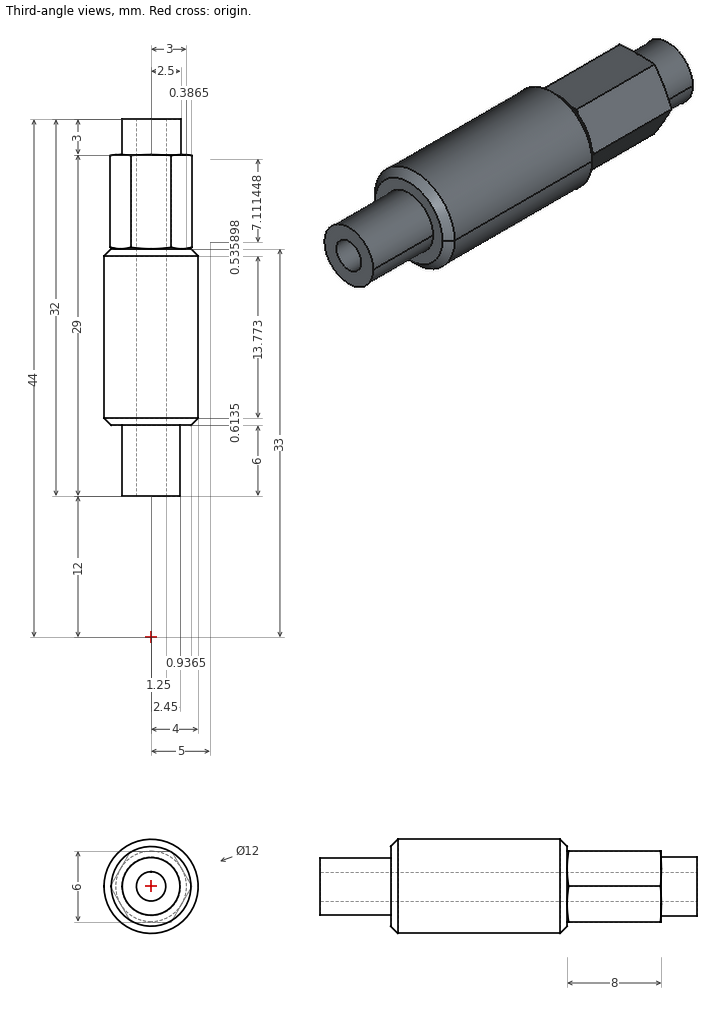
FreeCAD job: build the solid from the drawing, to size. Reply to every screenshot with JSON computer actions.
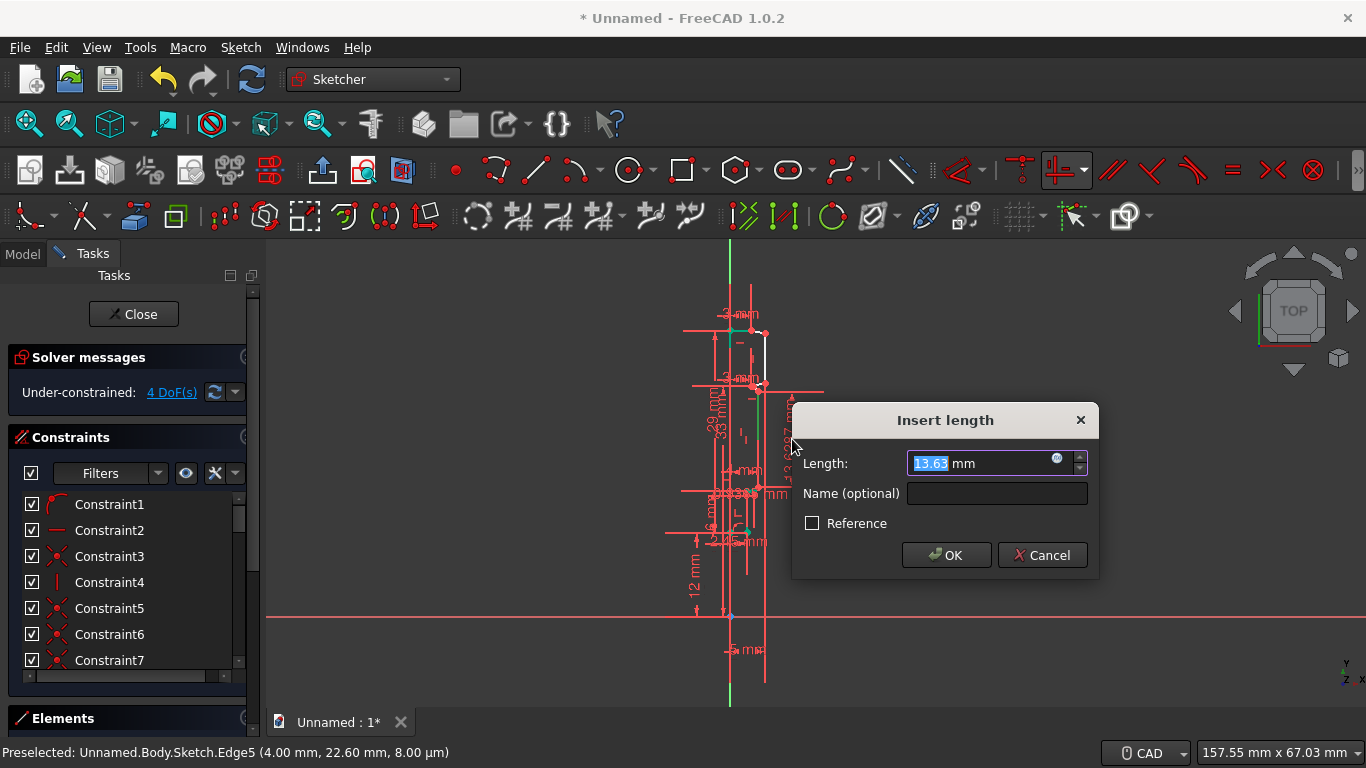
{"action": "type", "text": "13.773"}
{"action": "key", "text": "Return"}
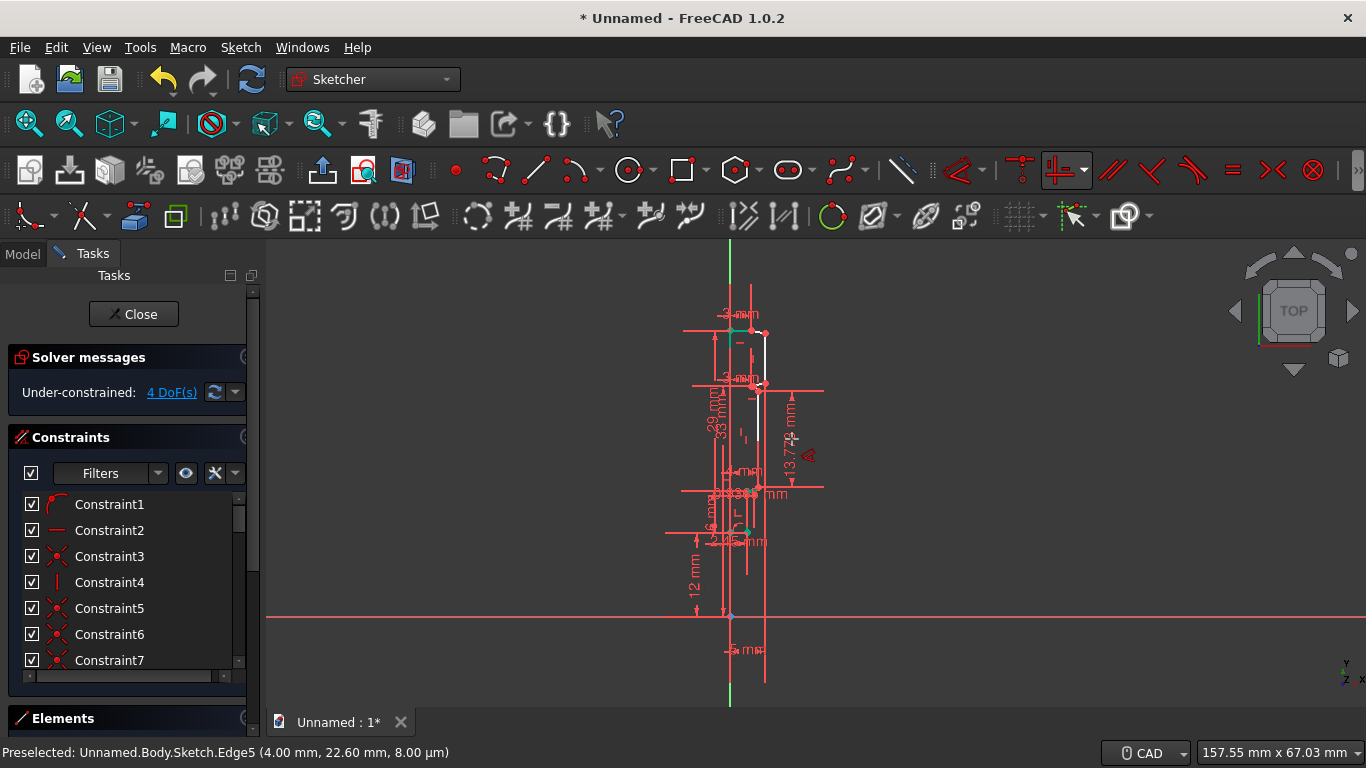
{"action": "scroll", "coordinate": [753, 386], "scroll_direction": "up", "scroll_amount": 14}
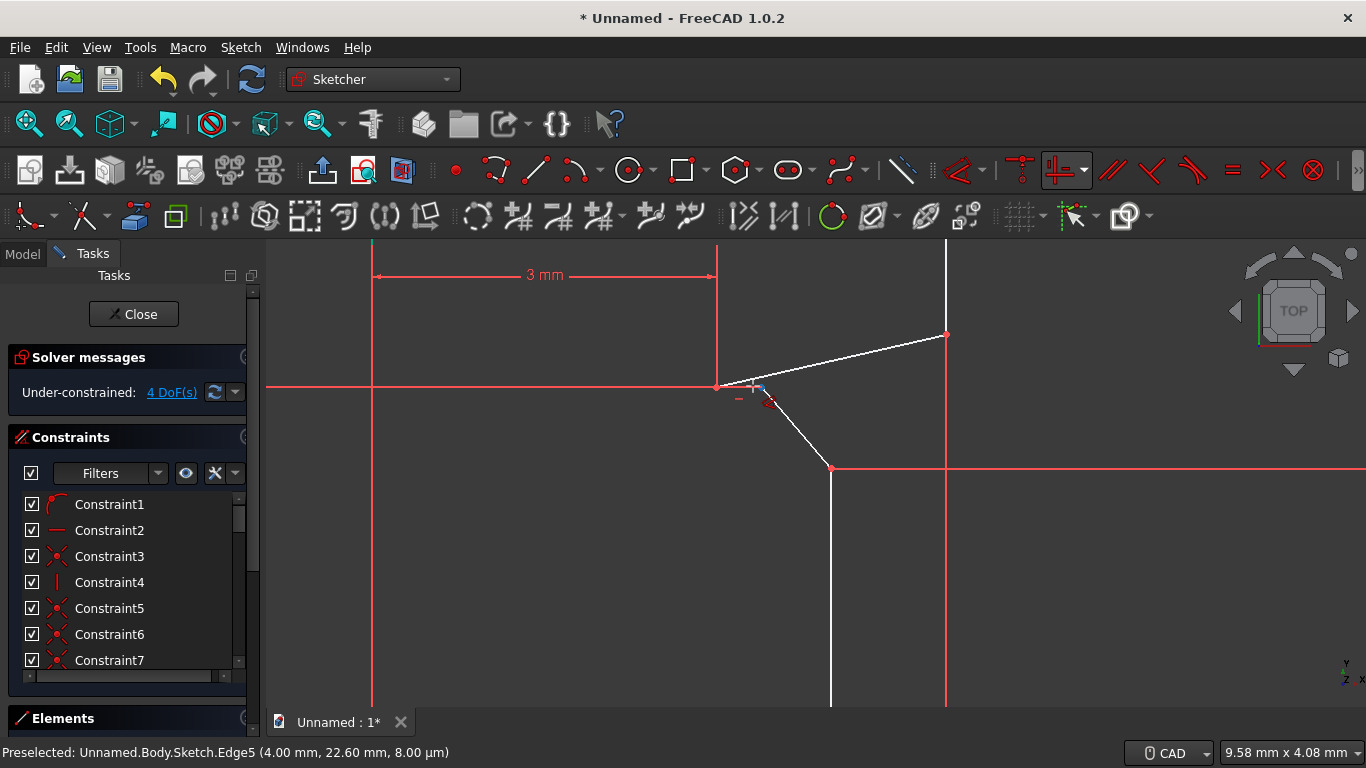
{"action": "left_click", "coordinate": [753, 387]}
{"action": "left_click", "coordinate": [739, 353]}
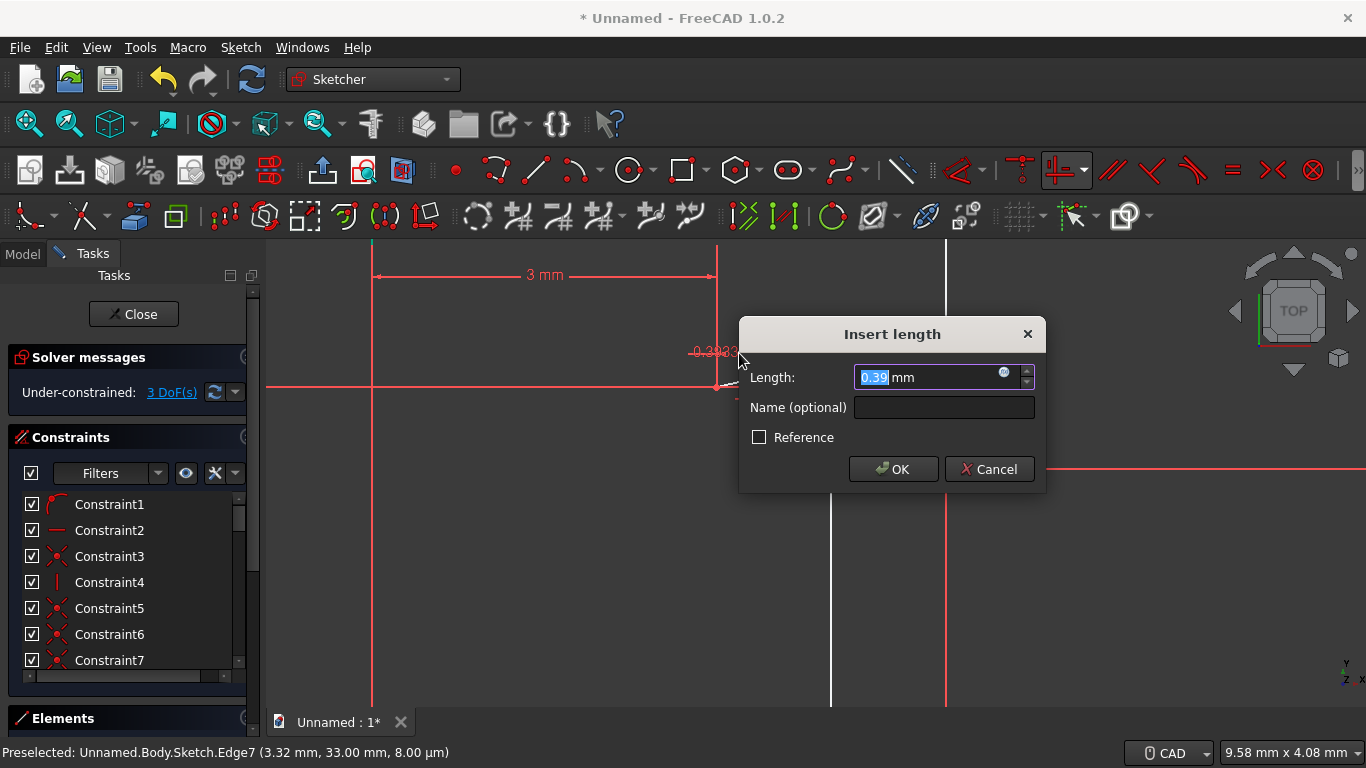
{"action": "type", "text": "0.3865"}
{"action": "key", "text": "Return"}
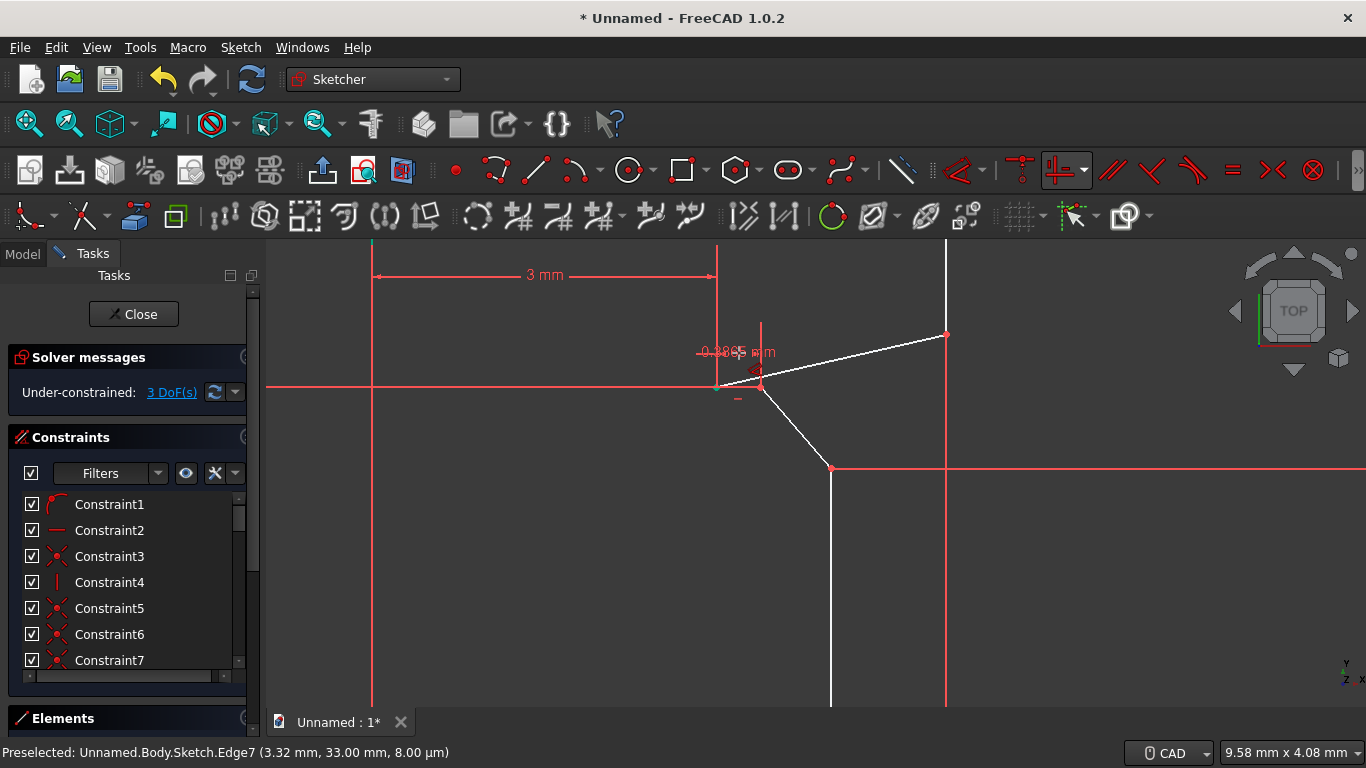
{"action": "scroll", "coordinate": [753, 386], "scroll_direction": "down", "scroll_amount": 14}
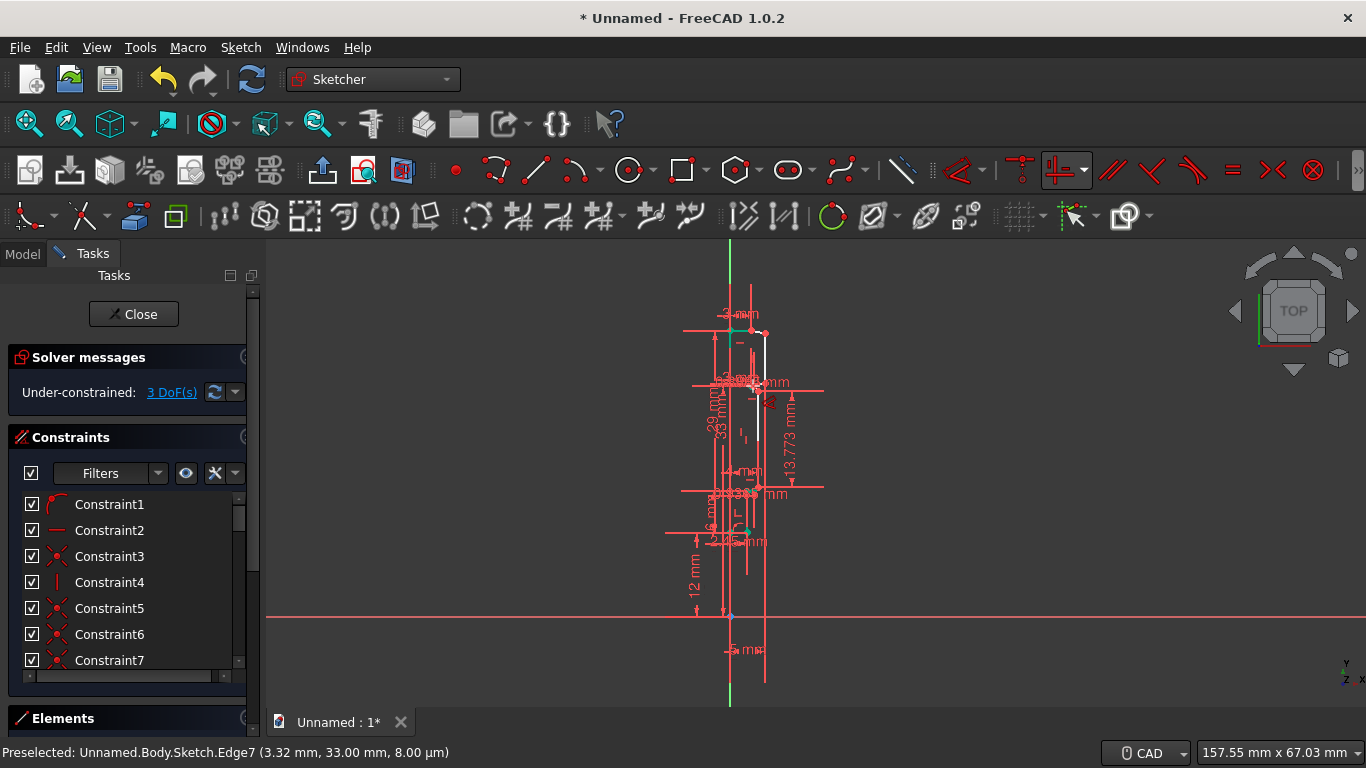
{"action": "scroll", "coordinate": [755, 490], "scroll_direction": "up", "scroll_amount": 12}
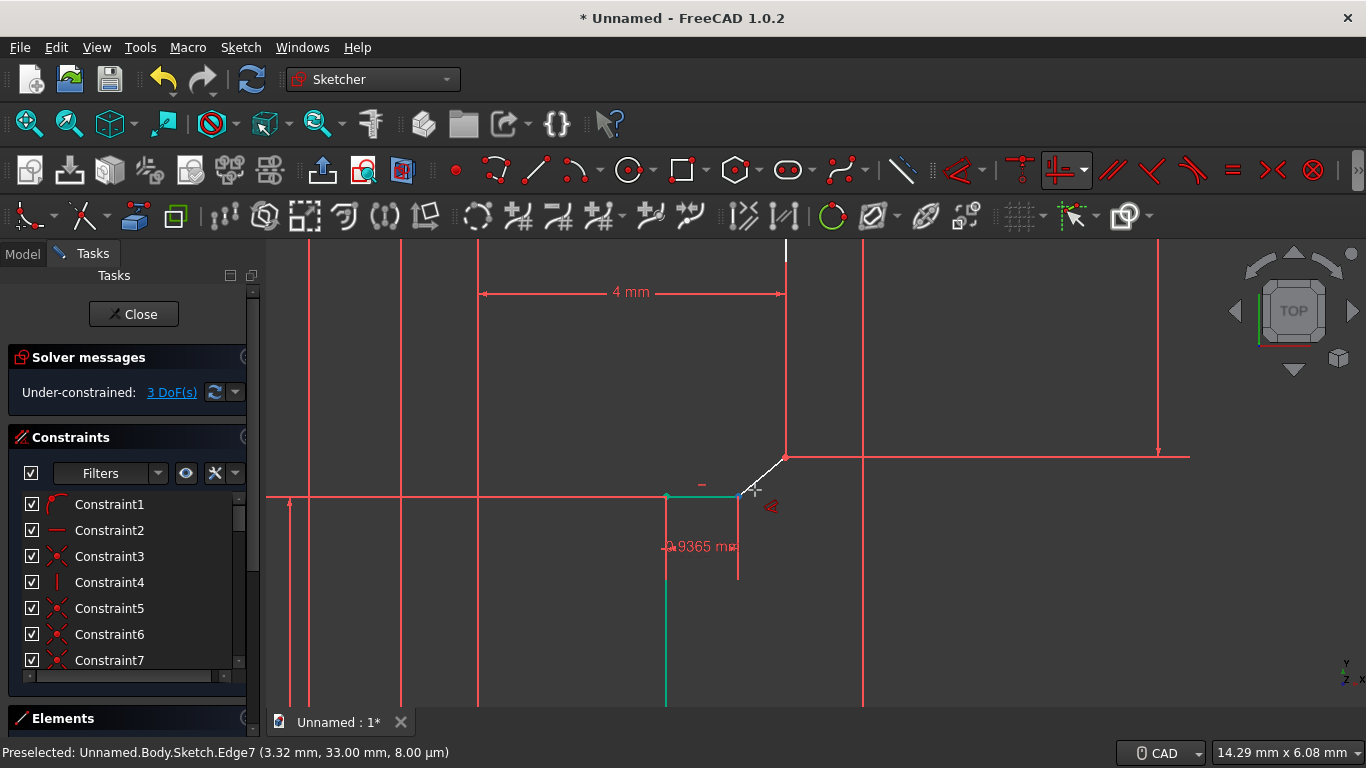
{"action": "left_click", "coordinate": [753, 485]}
{"action": "left_click", "coordinate": [820, 477]}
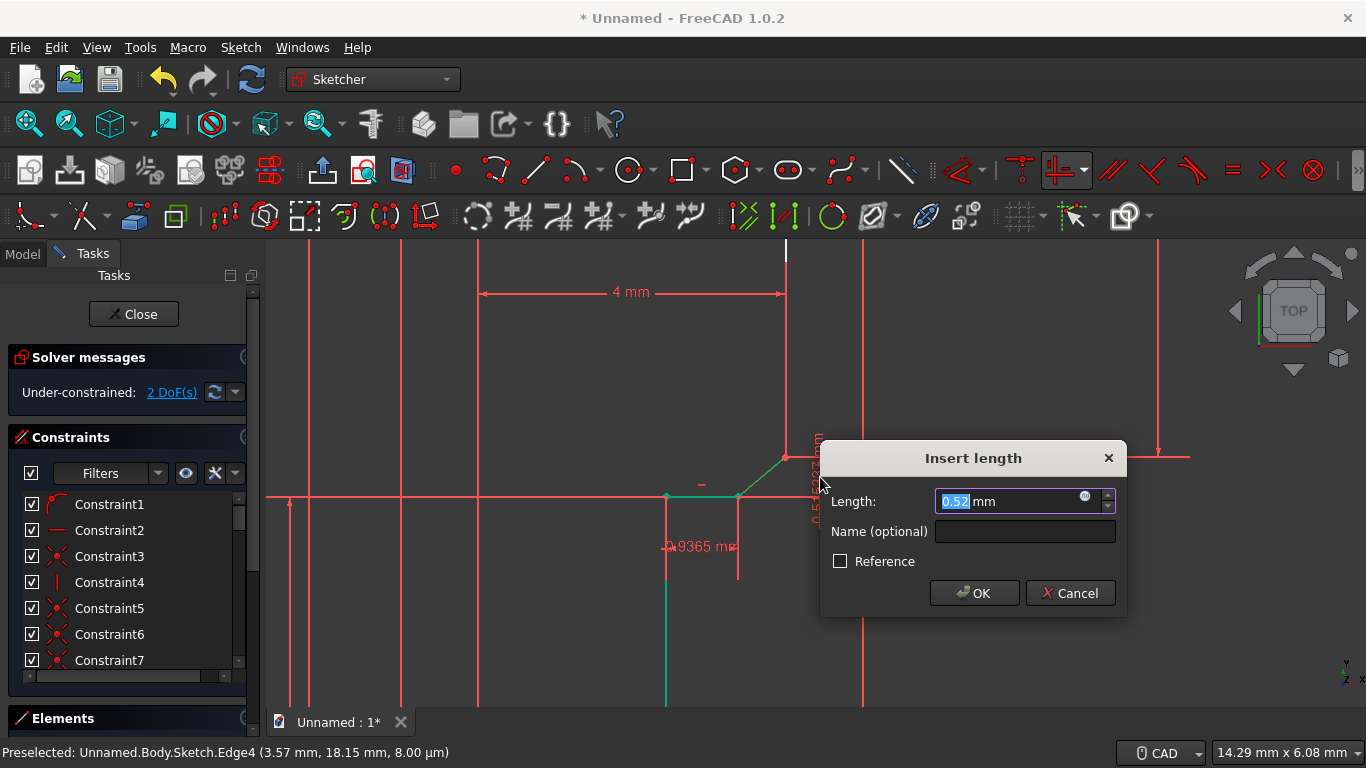
{"action": "type", "text": "0.6135"}
{"action": "key", "text": "Return"}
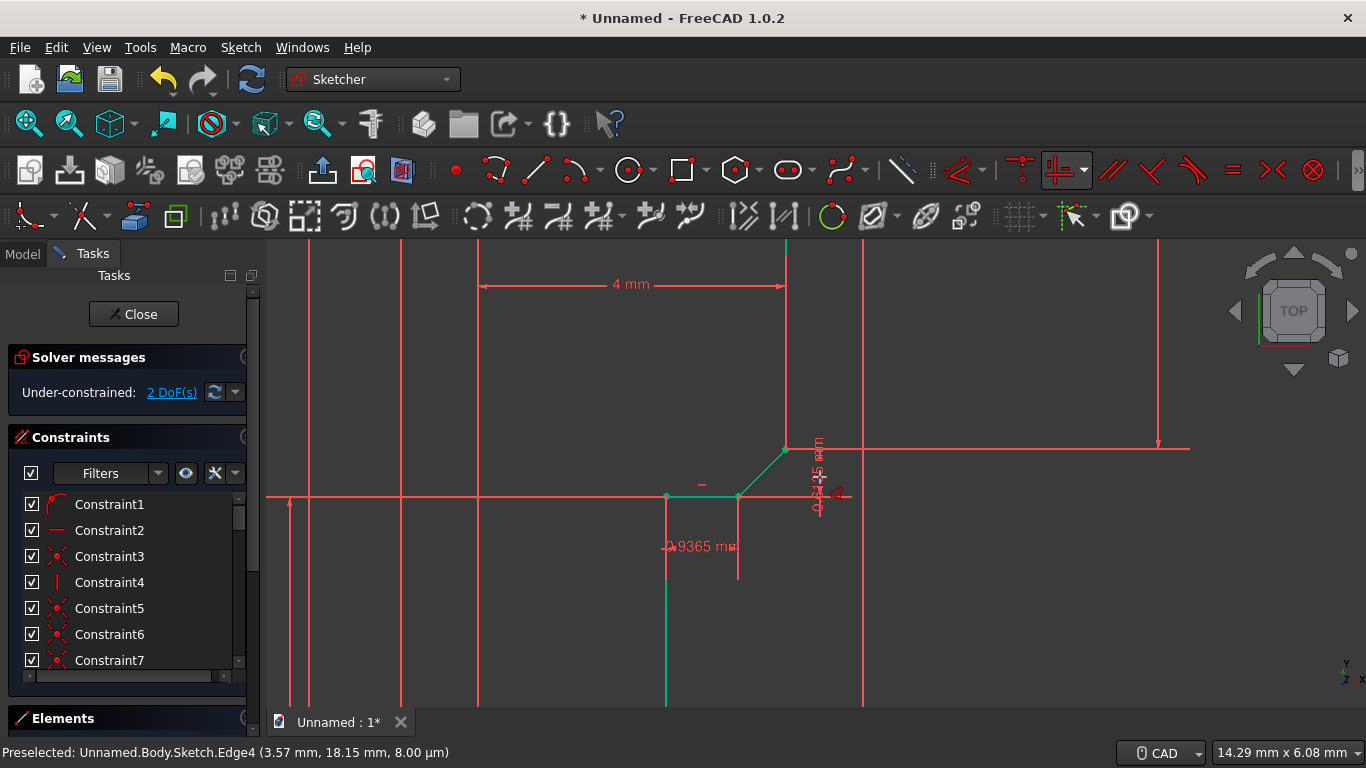
{"action": "scroll", "coordinate": [755, 490], "scroll_direction": "down", "scroll_amount": 12}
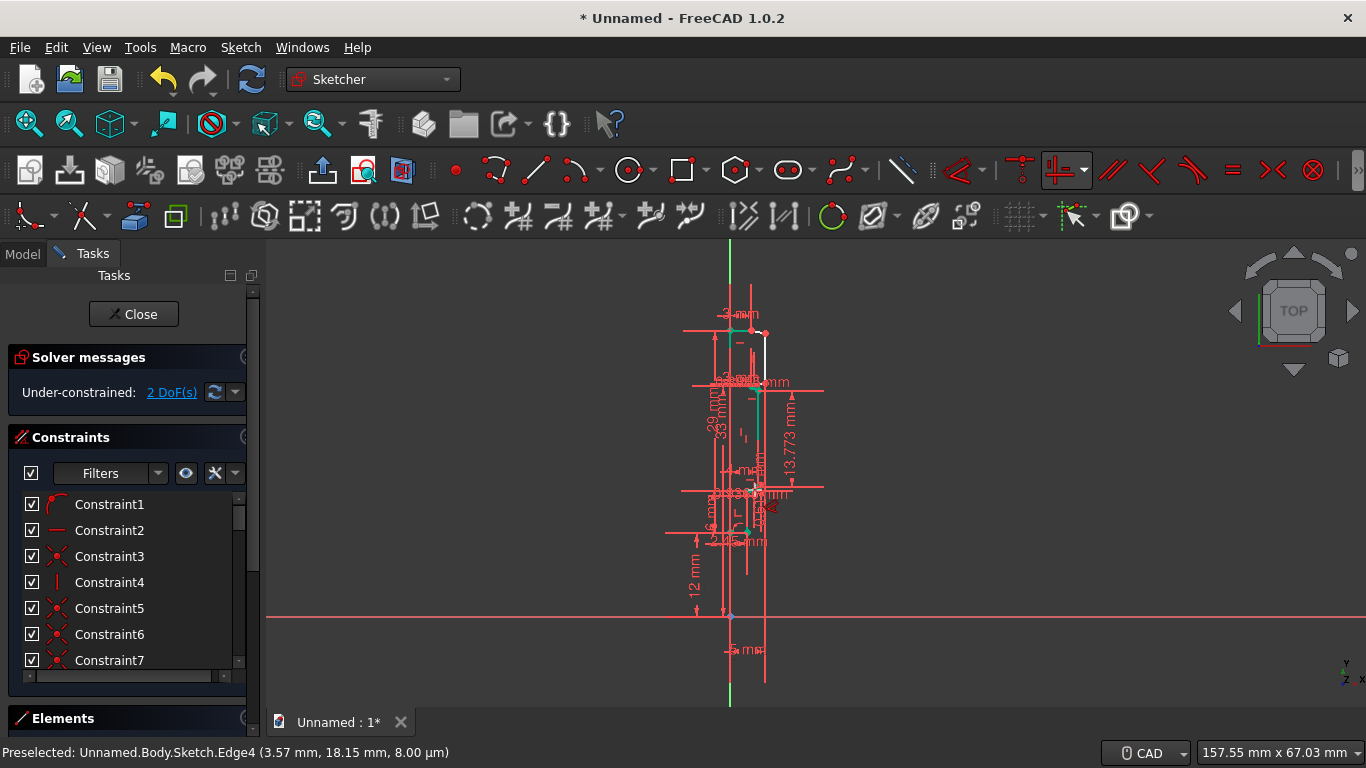
{"action": "left_click", "coordinate": [765, 368]}
{"action": "left_click", "coordinate": [799, 358]}